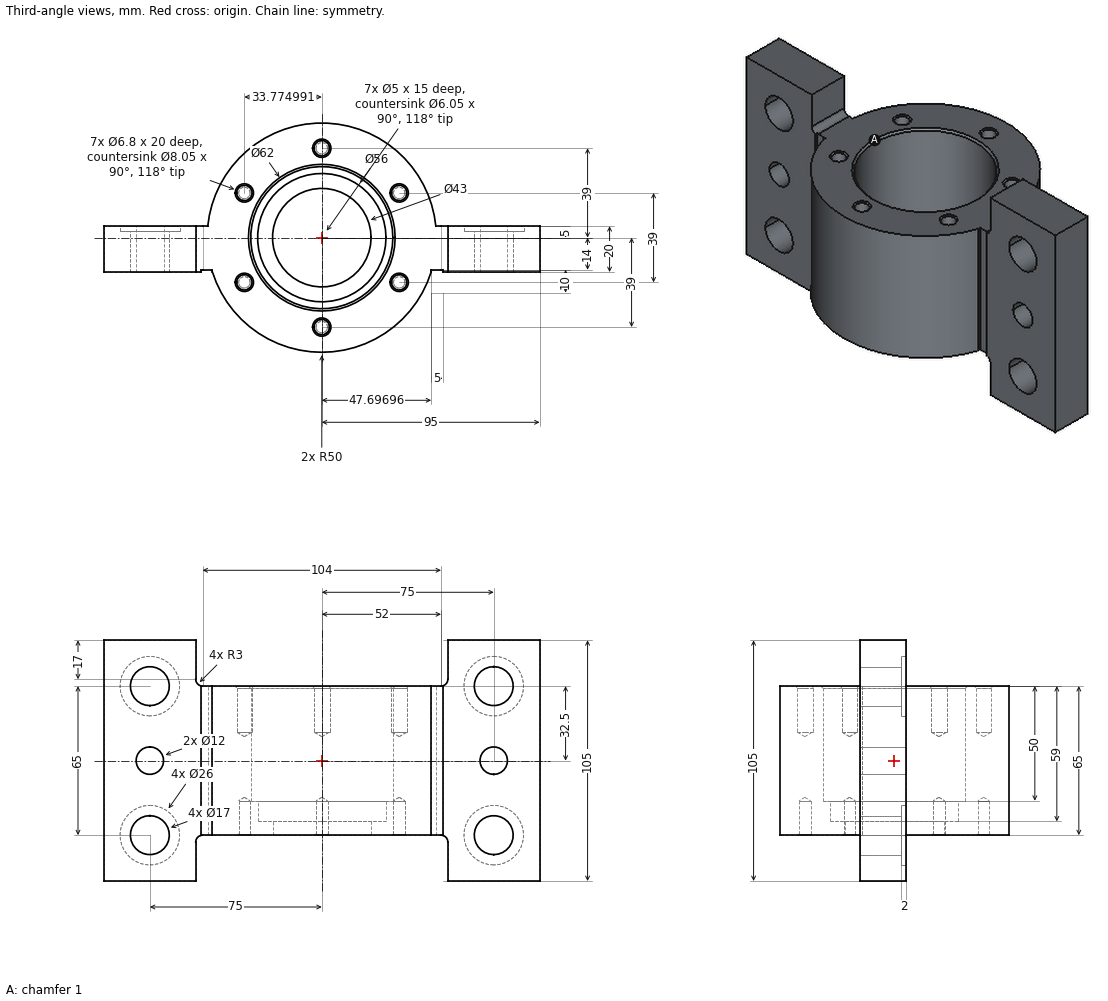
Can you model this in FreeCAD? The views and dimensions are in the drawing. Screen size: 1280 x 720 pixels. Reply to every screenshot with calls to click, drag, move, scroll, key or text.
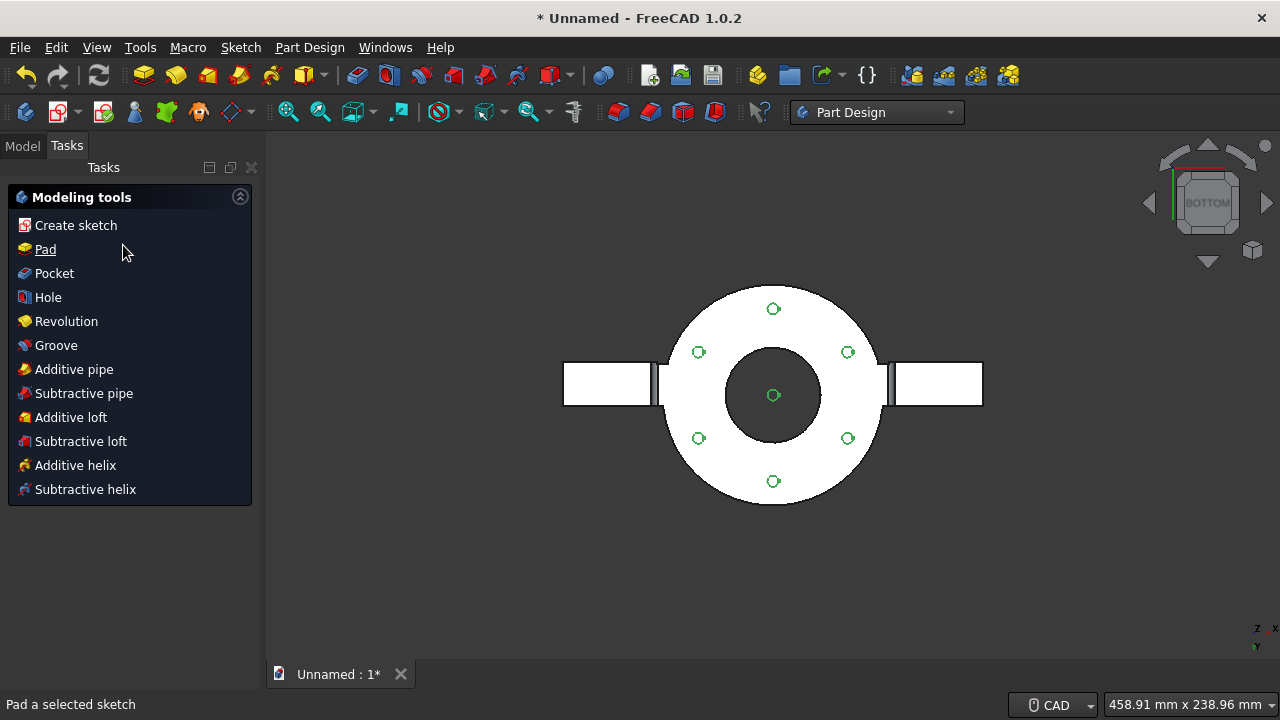
click(390, 76)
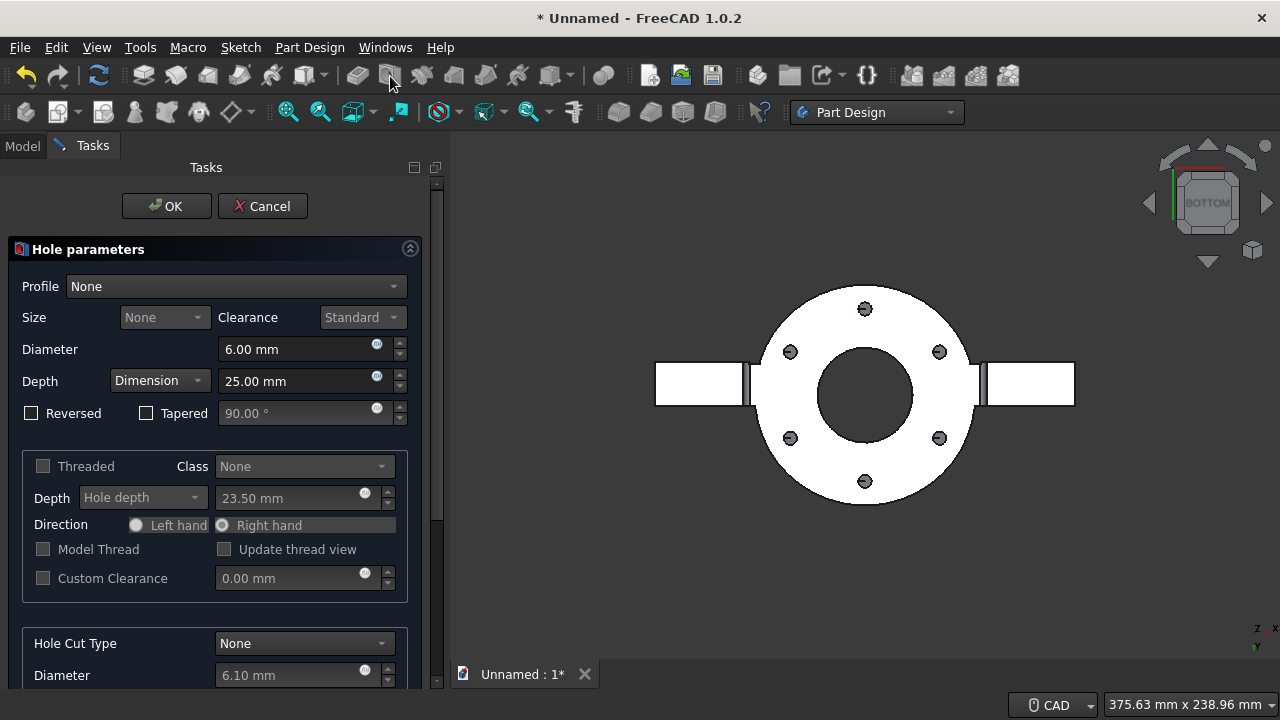
triple_click(305, 349)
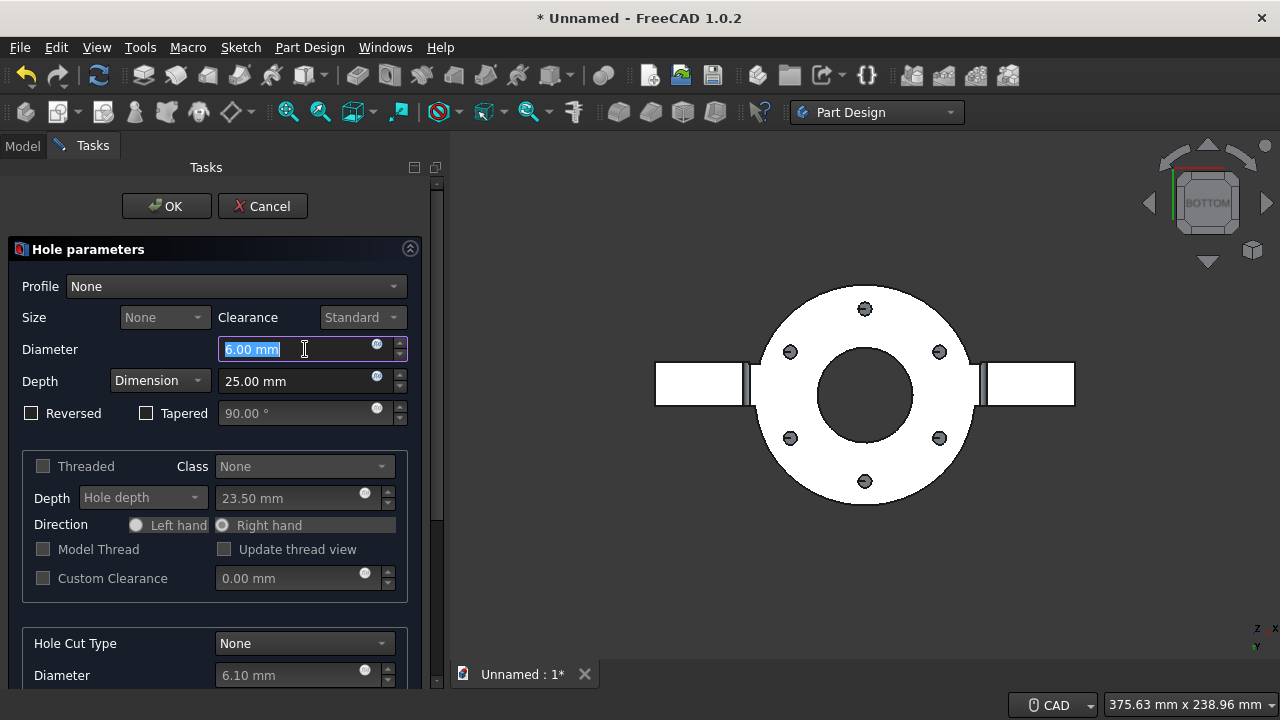
text(5)
key(Tab)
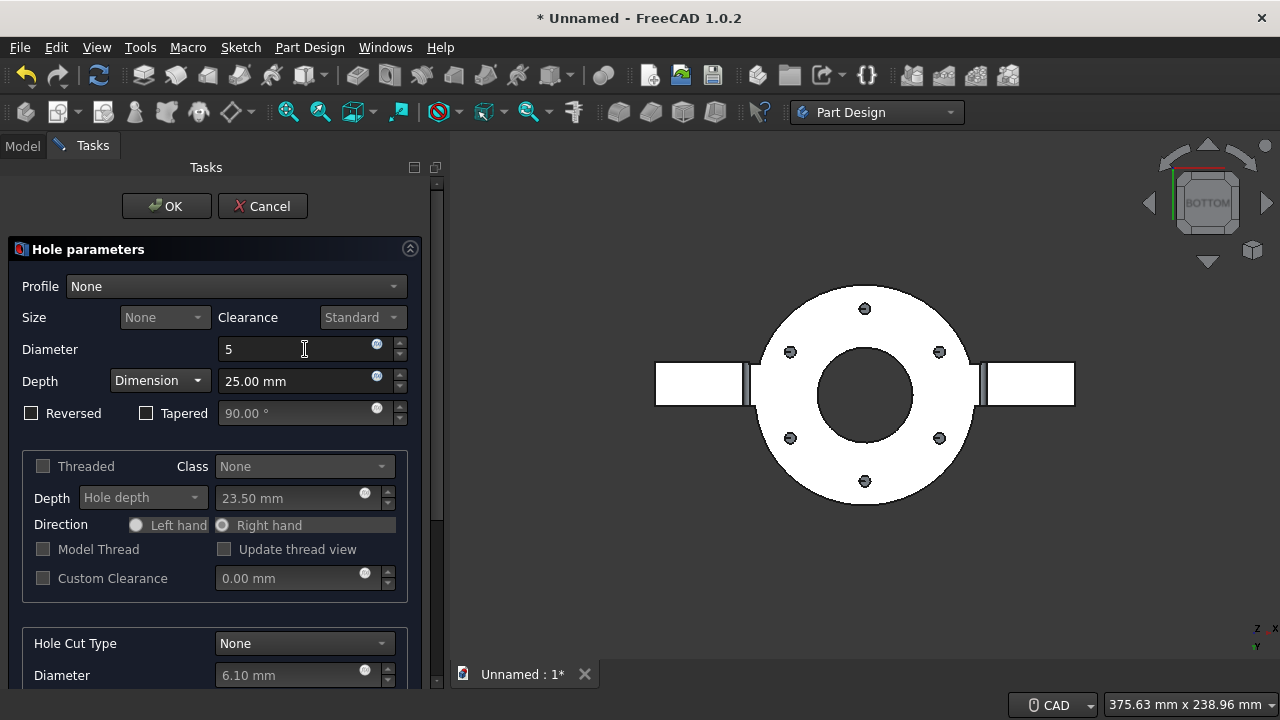
triple_click(305, 381)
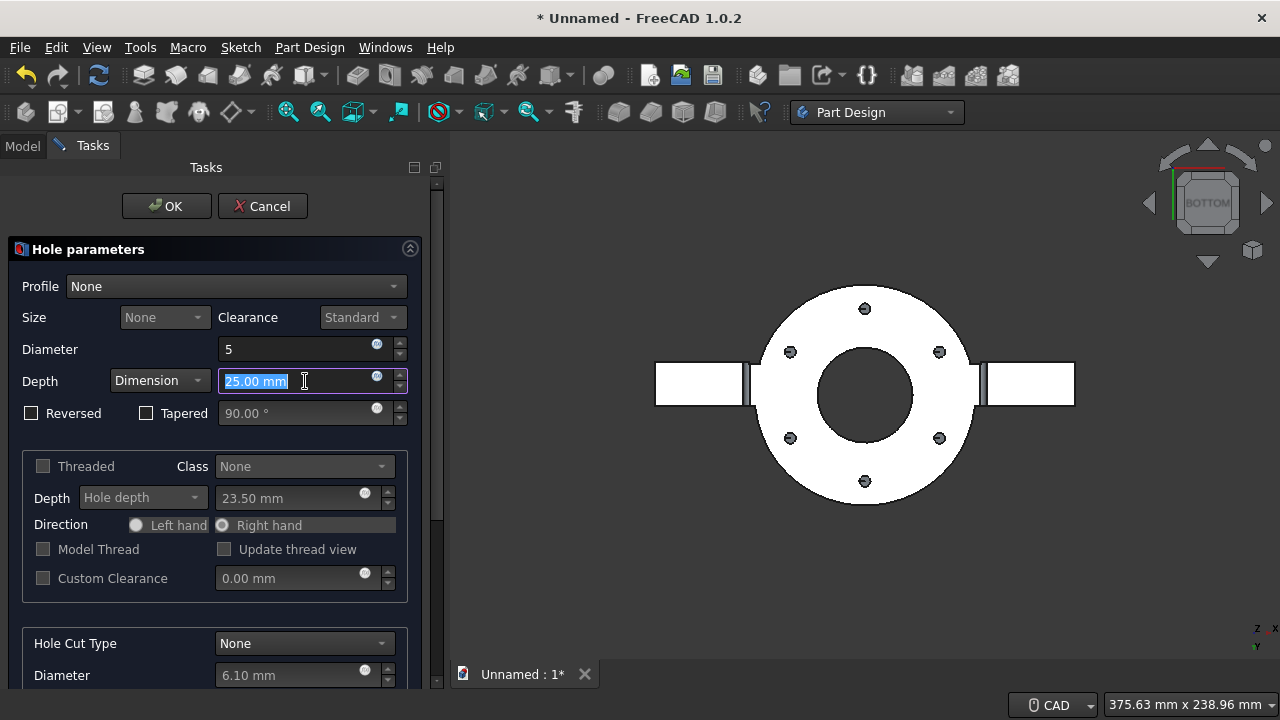
text(15)
key(Tab)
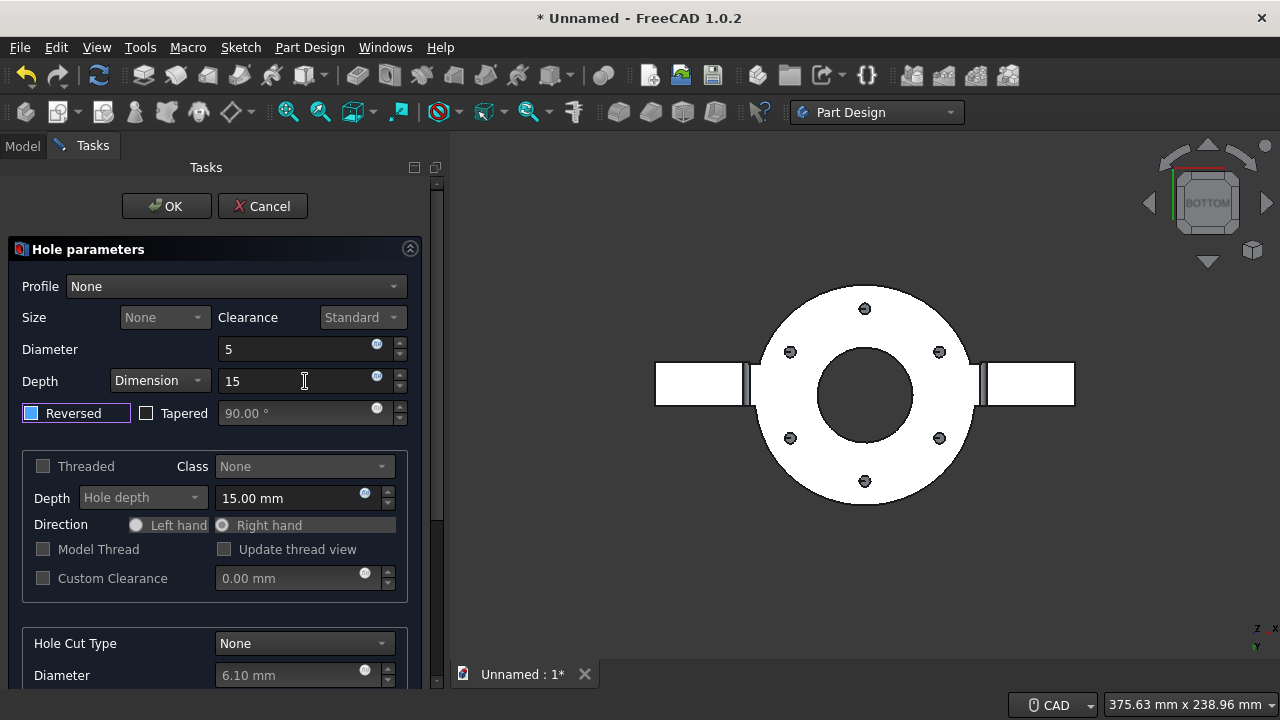
click(306, 644)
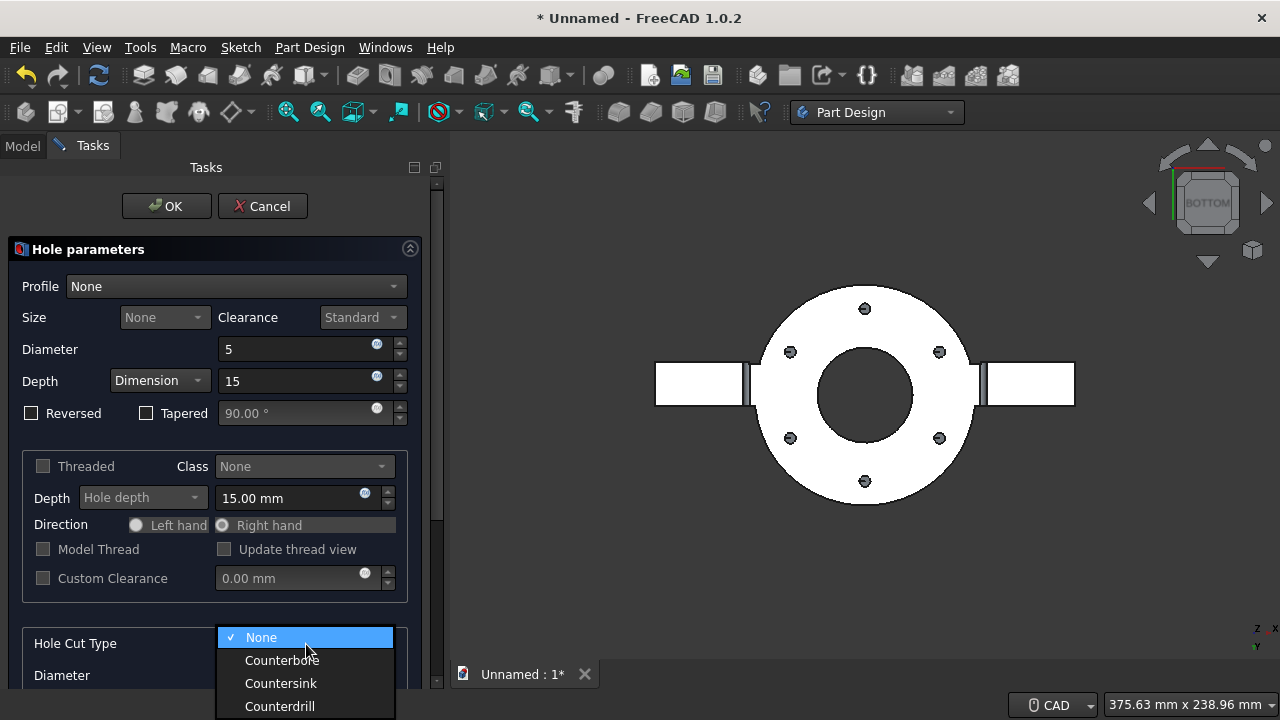
click(304, 684)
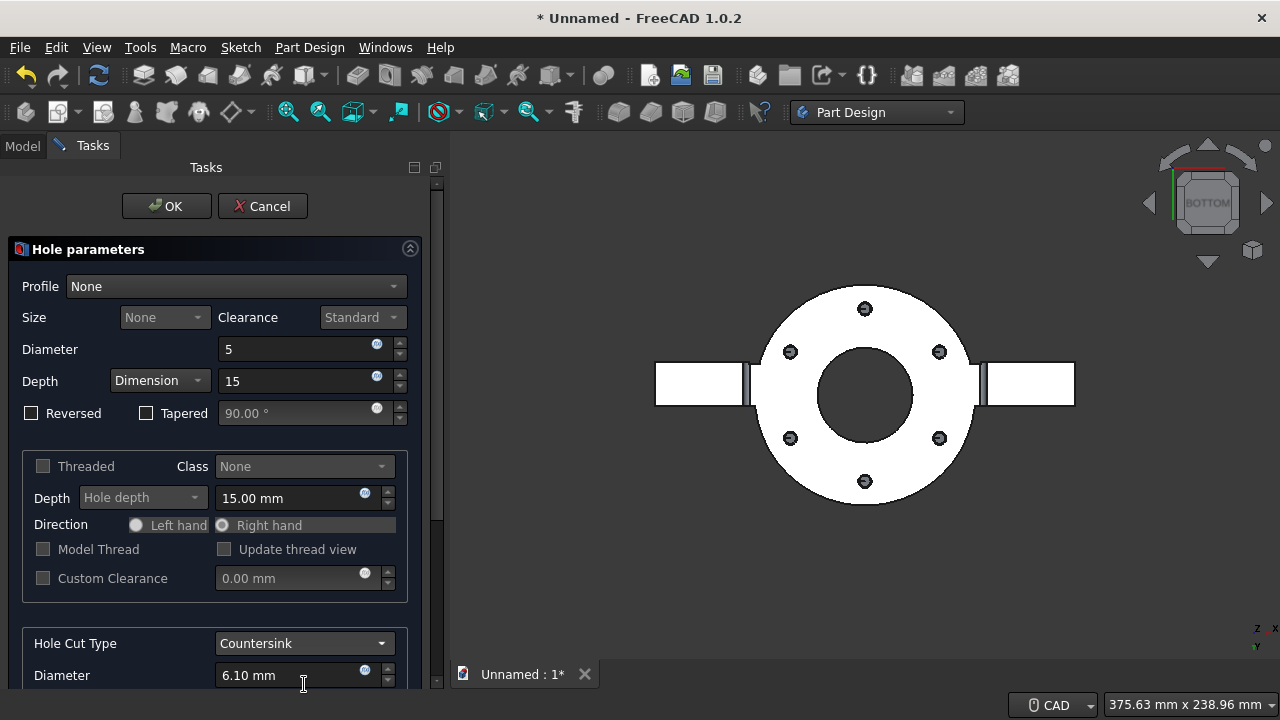
triple_click(298, 675)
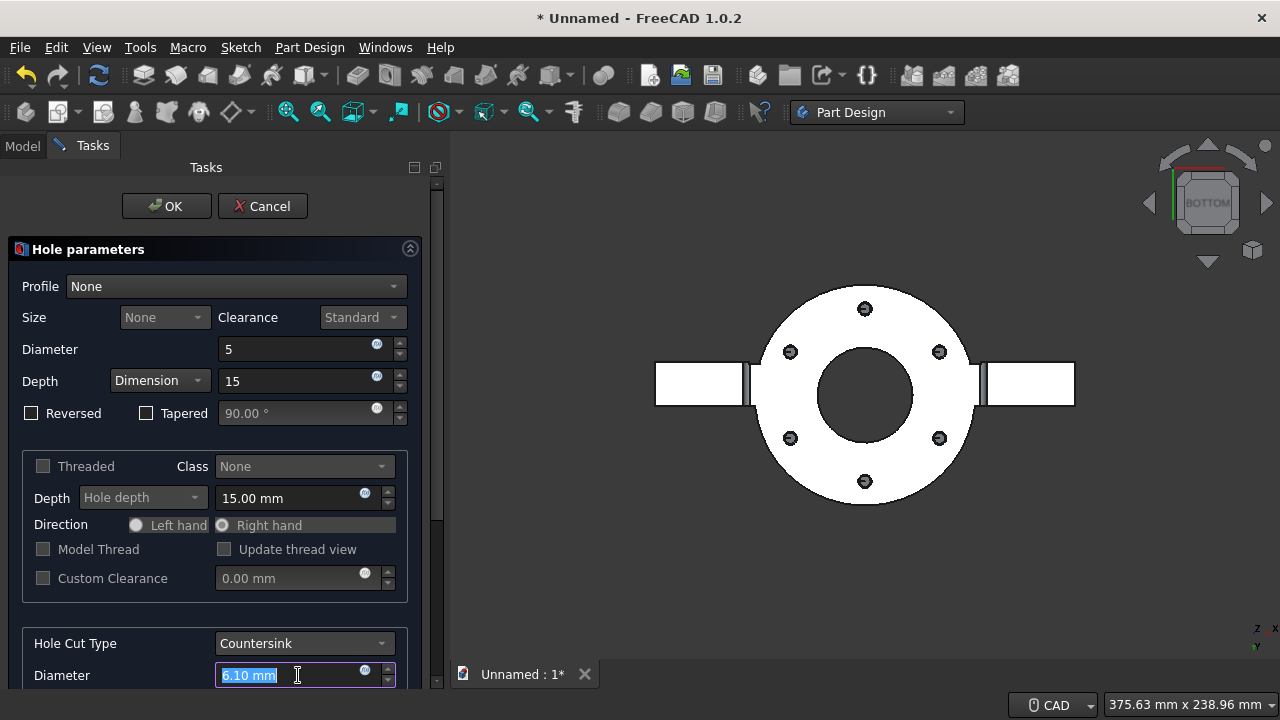
text(6.05)
key(Tab)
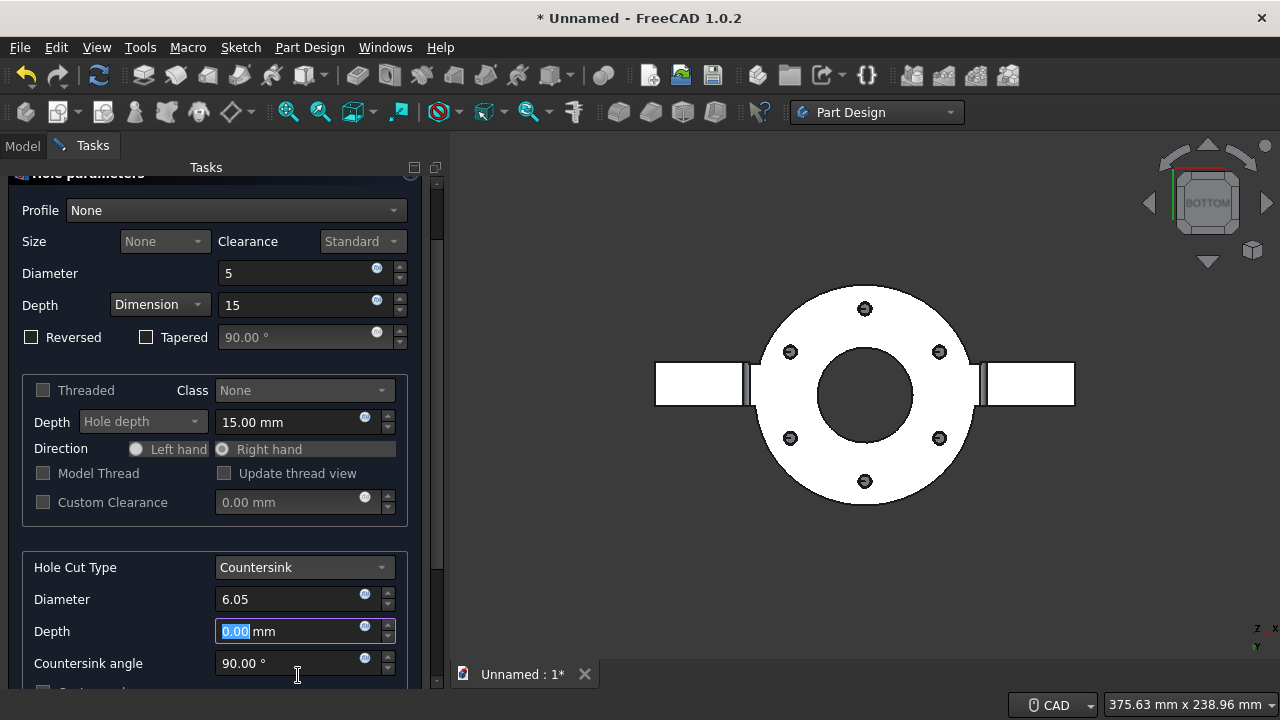
scroll(437, 432, up, 3)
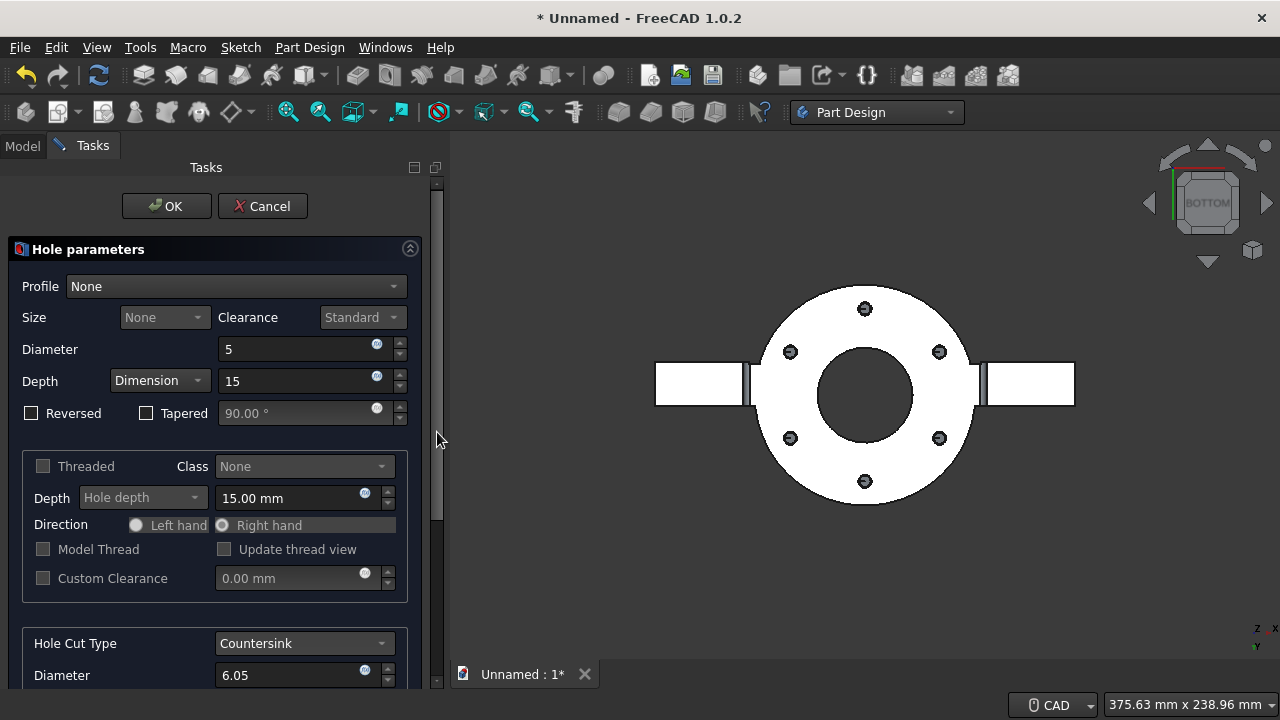
click(167, 206)